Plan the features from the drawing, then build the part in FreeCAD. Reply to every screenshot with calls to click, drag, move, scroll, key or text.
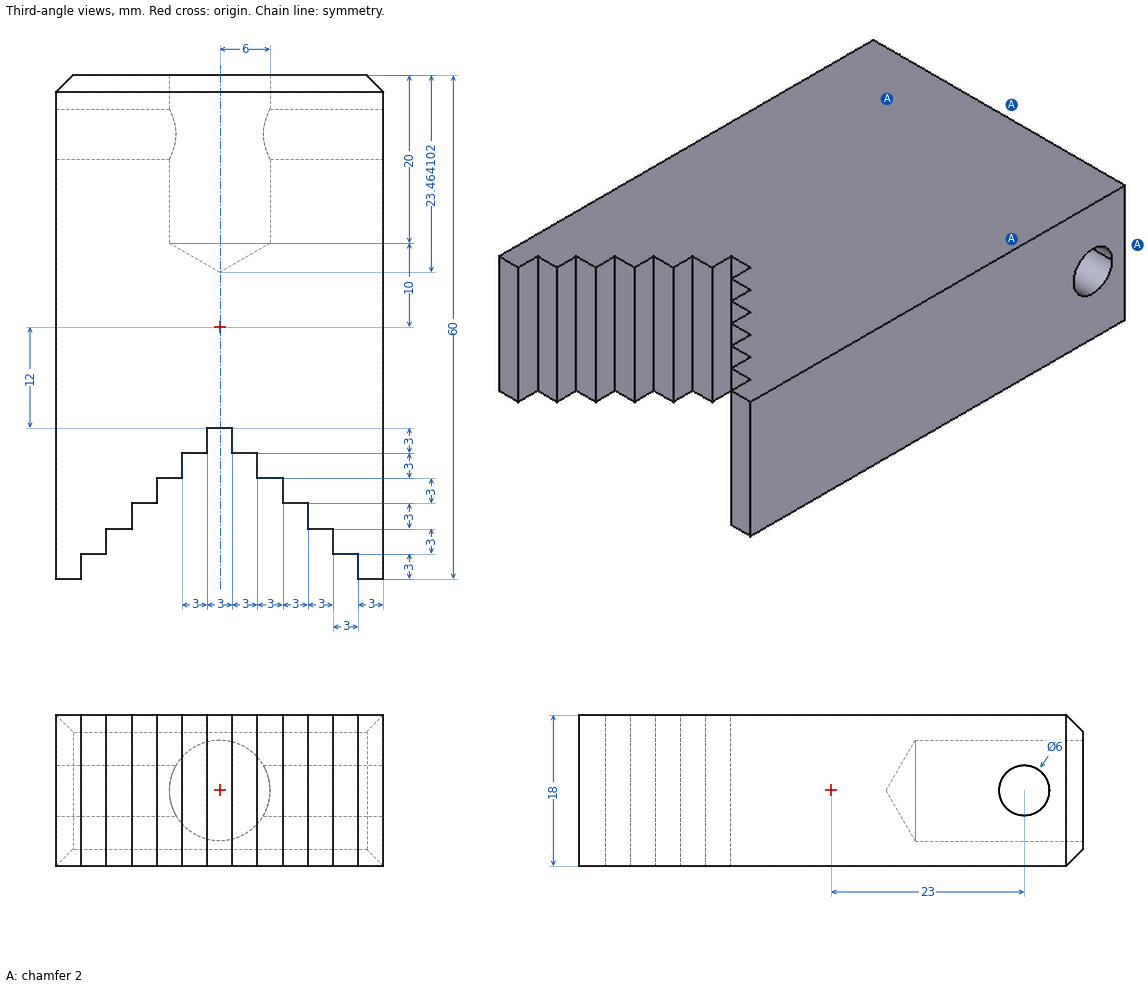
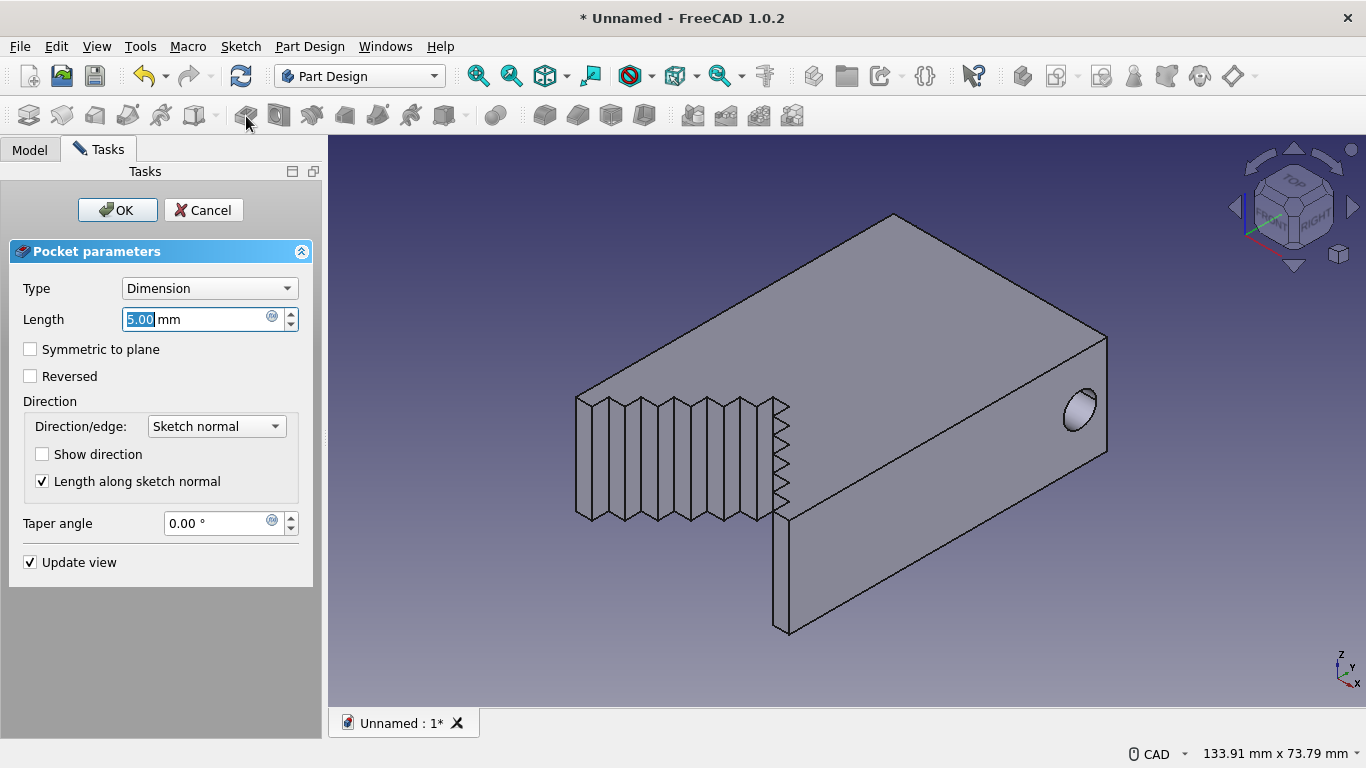
click(210, 288)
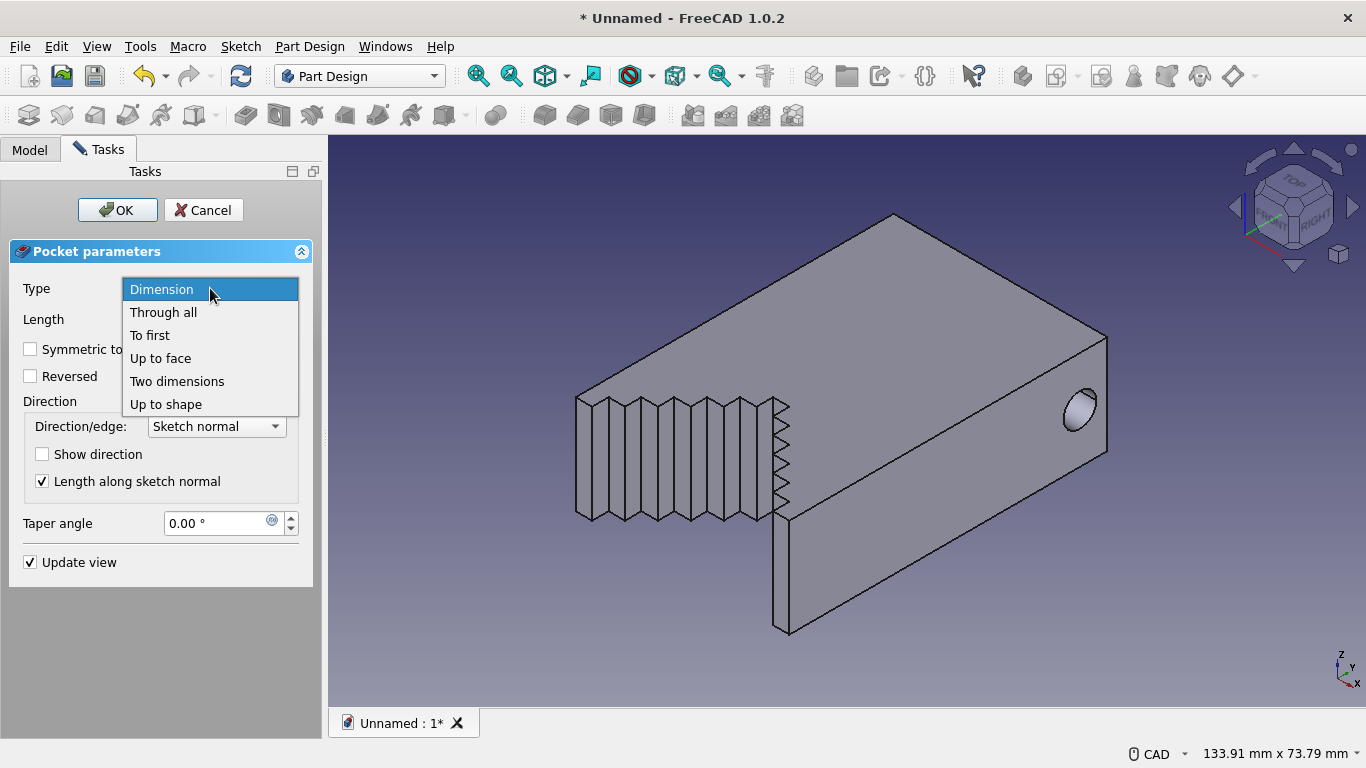
click(208, 312)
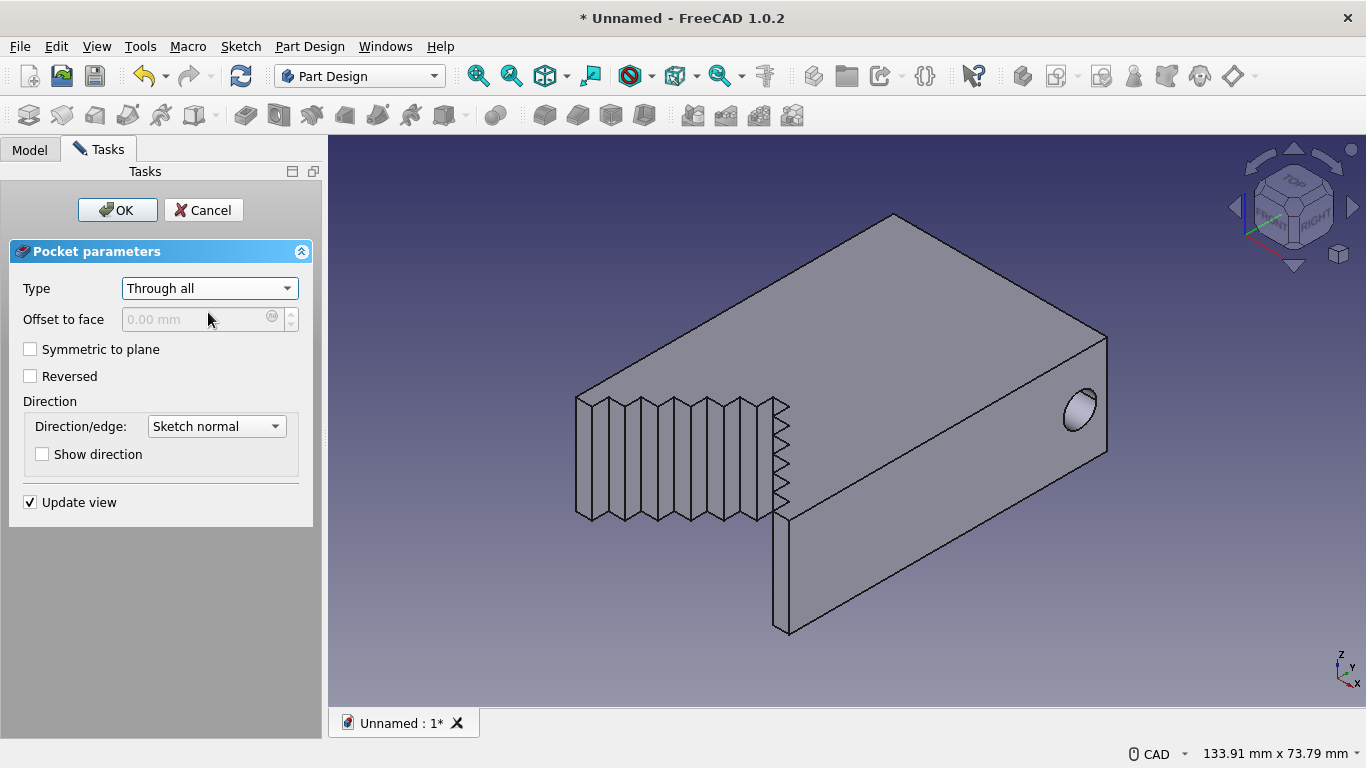
click(118, 210)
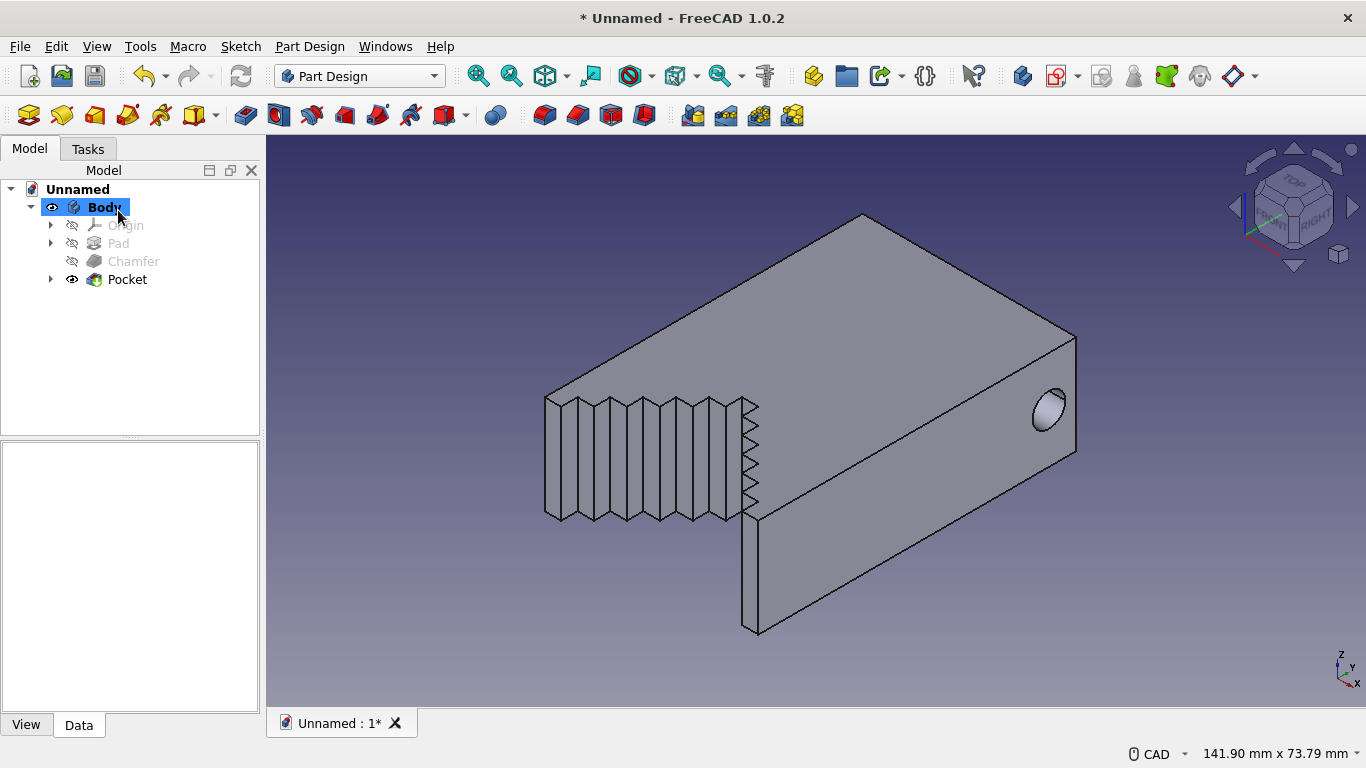
click(1056, 76)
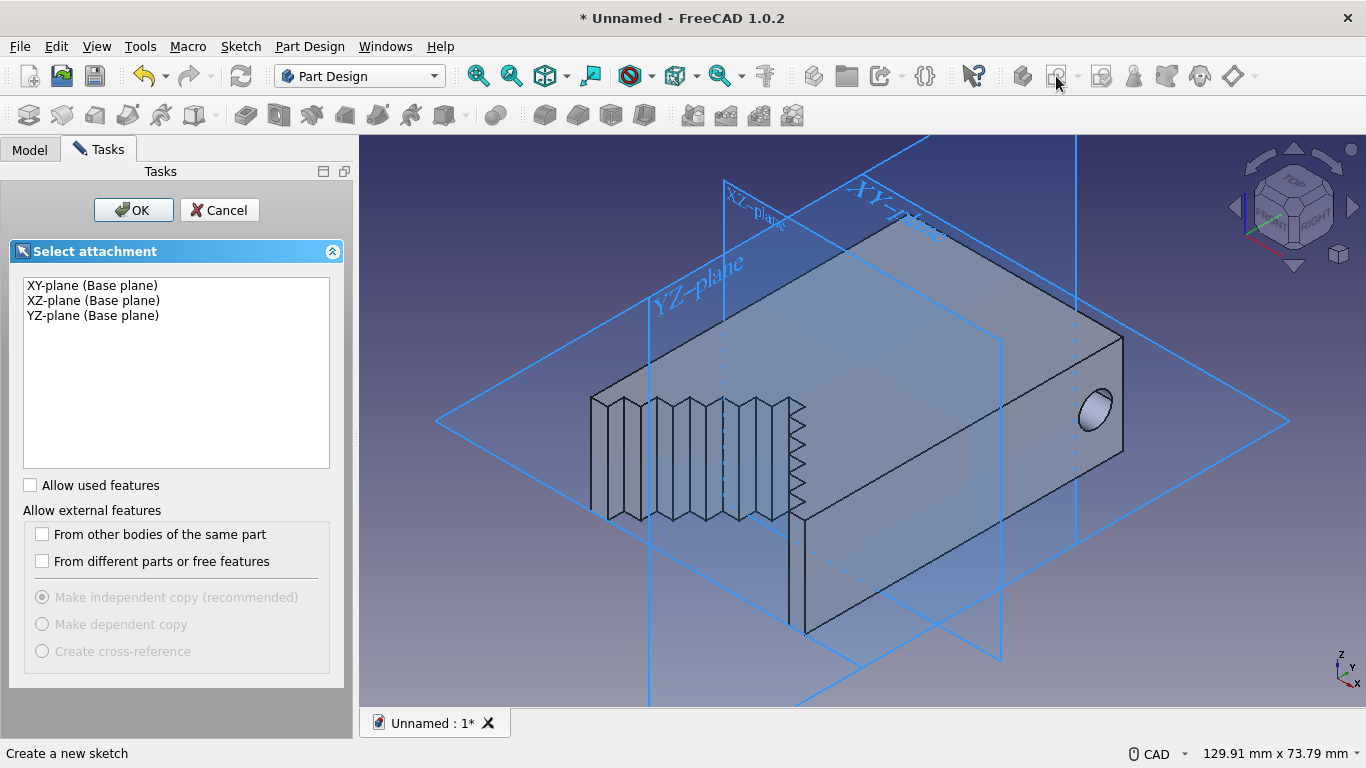
click(84, 286)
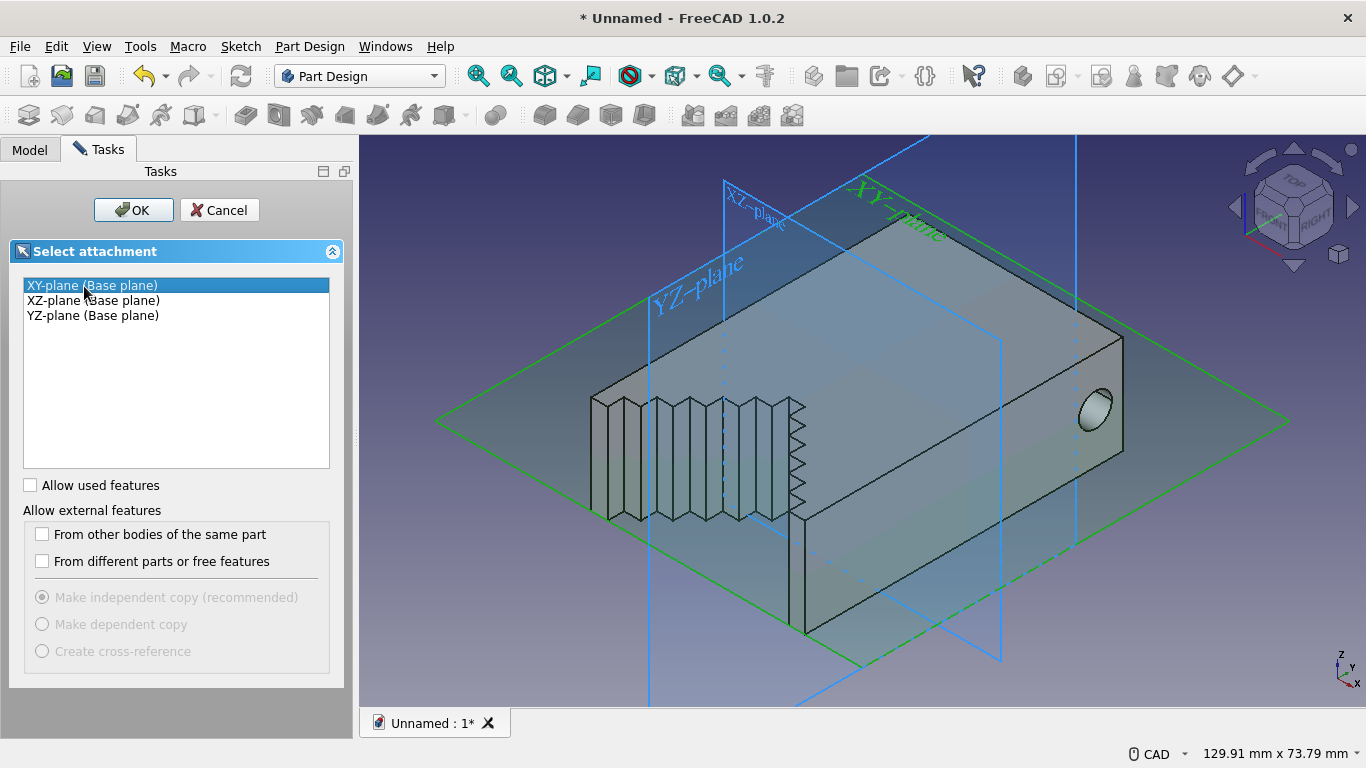
click(134, 210)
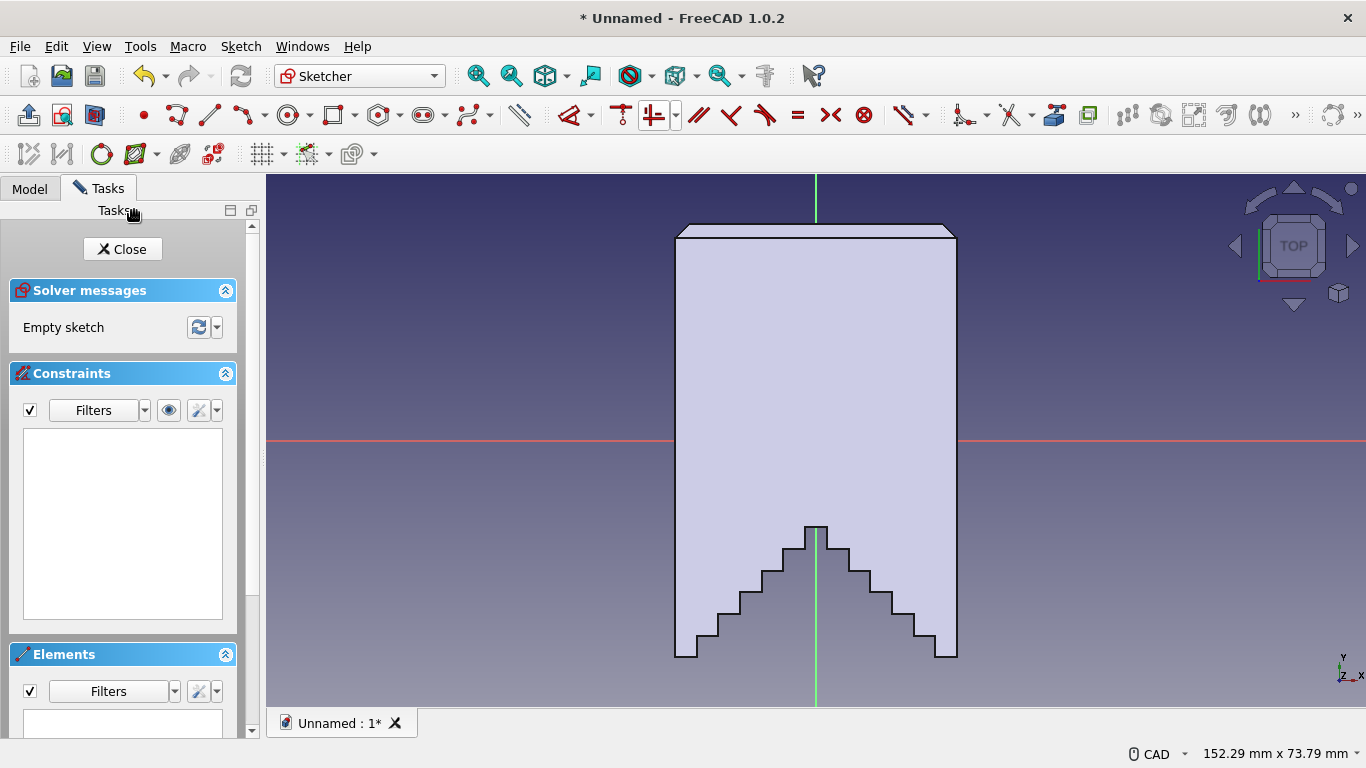
click(95, 116)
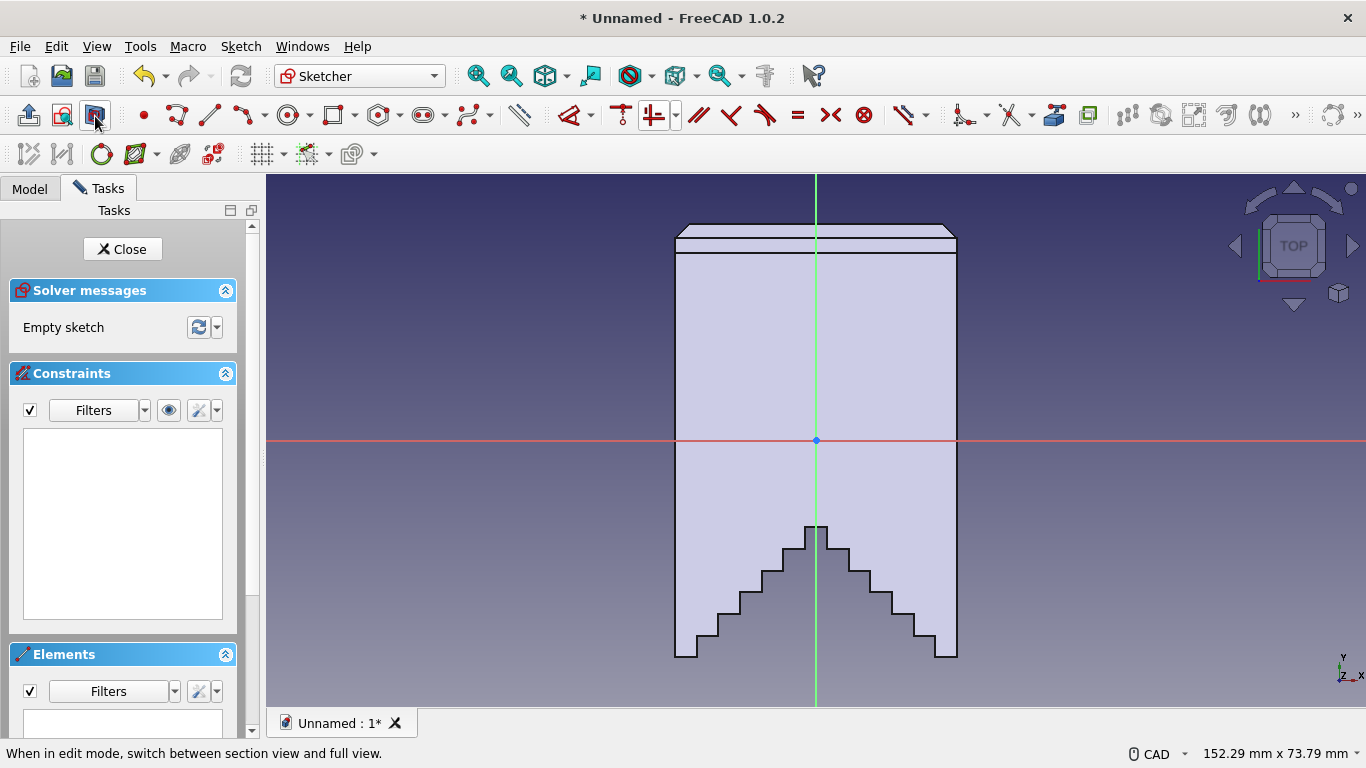
scroll(1021, 202, up, 2)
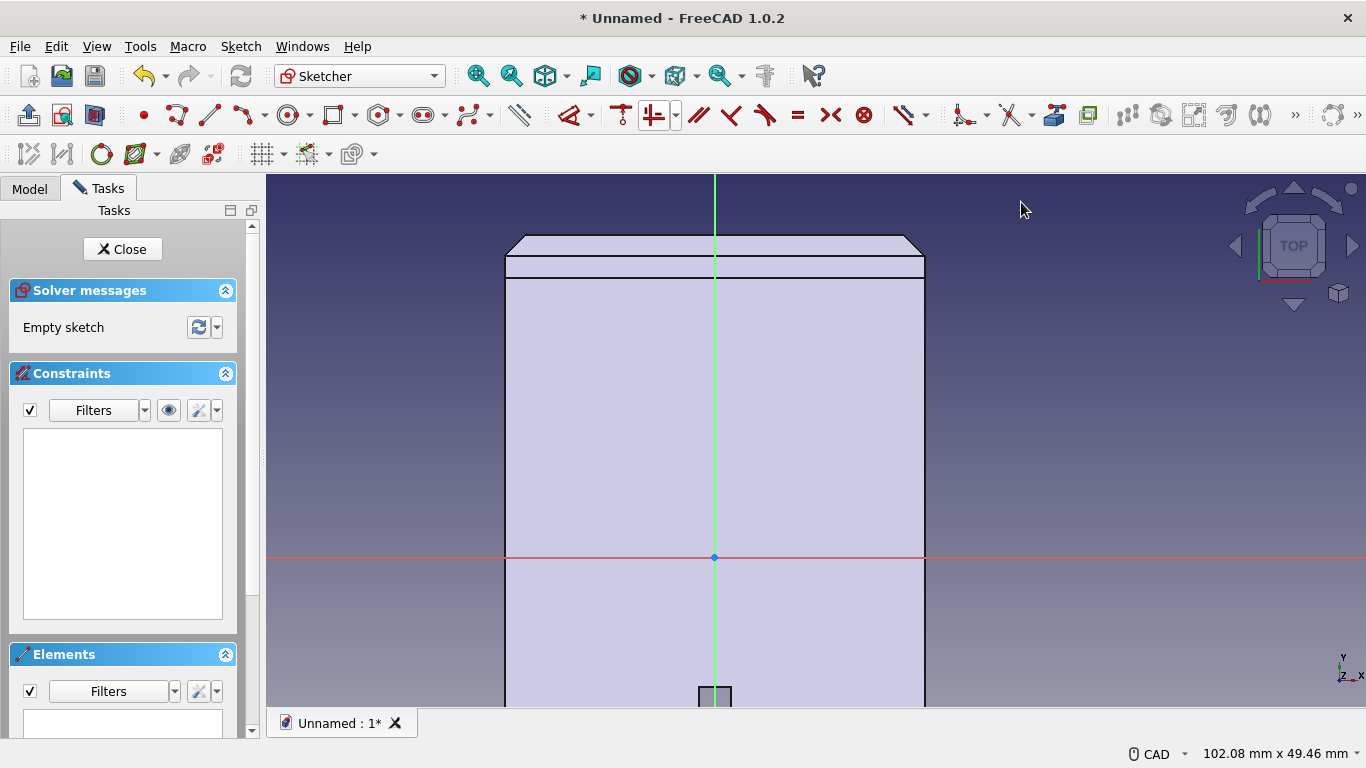
click(177, 116)